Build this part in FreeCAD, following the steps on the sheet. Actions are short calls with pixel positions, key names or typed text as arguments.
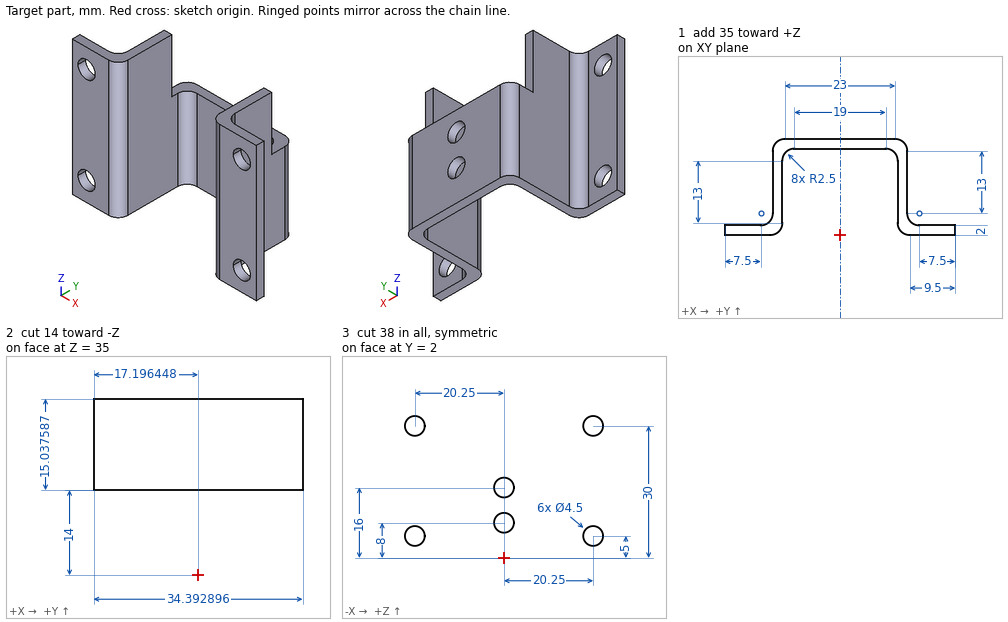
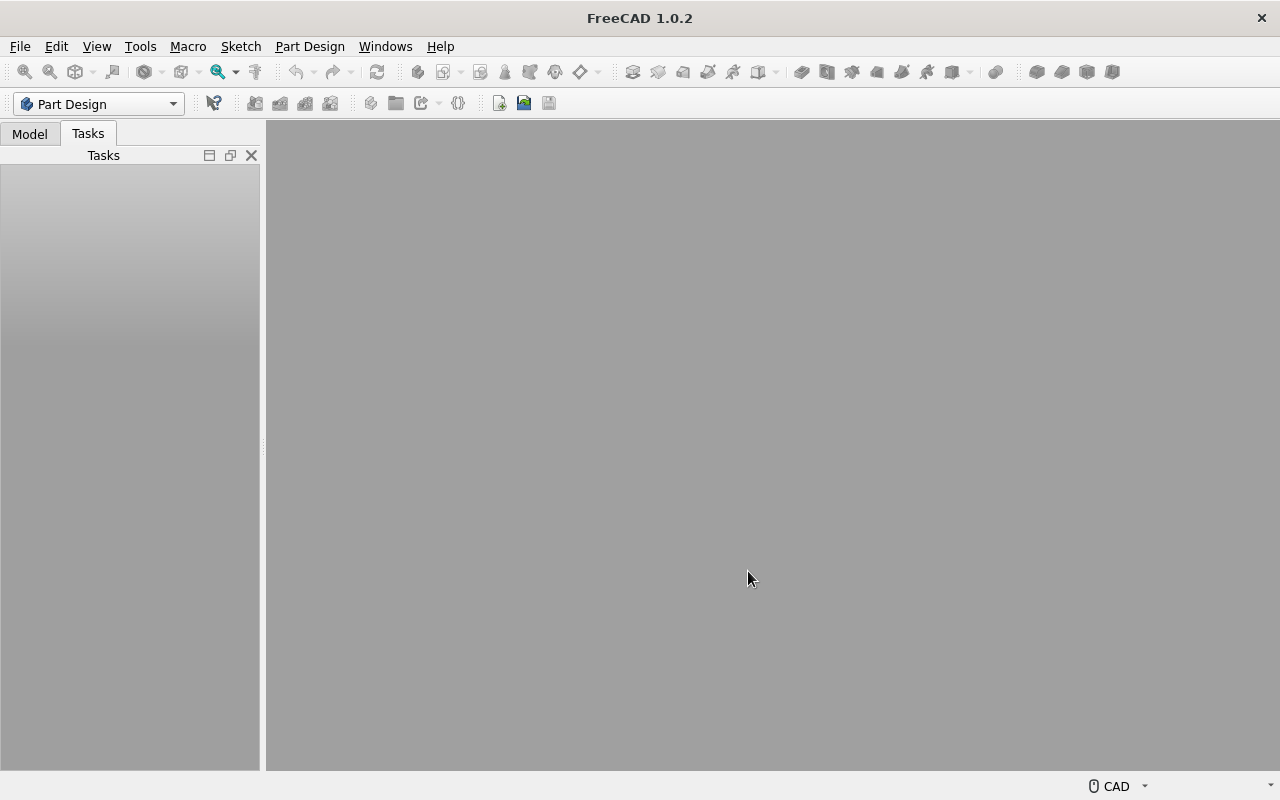
key(ctrl+n)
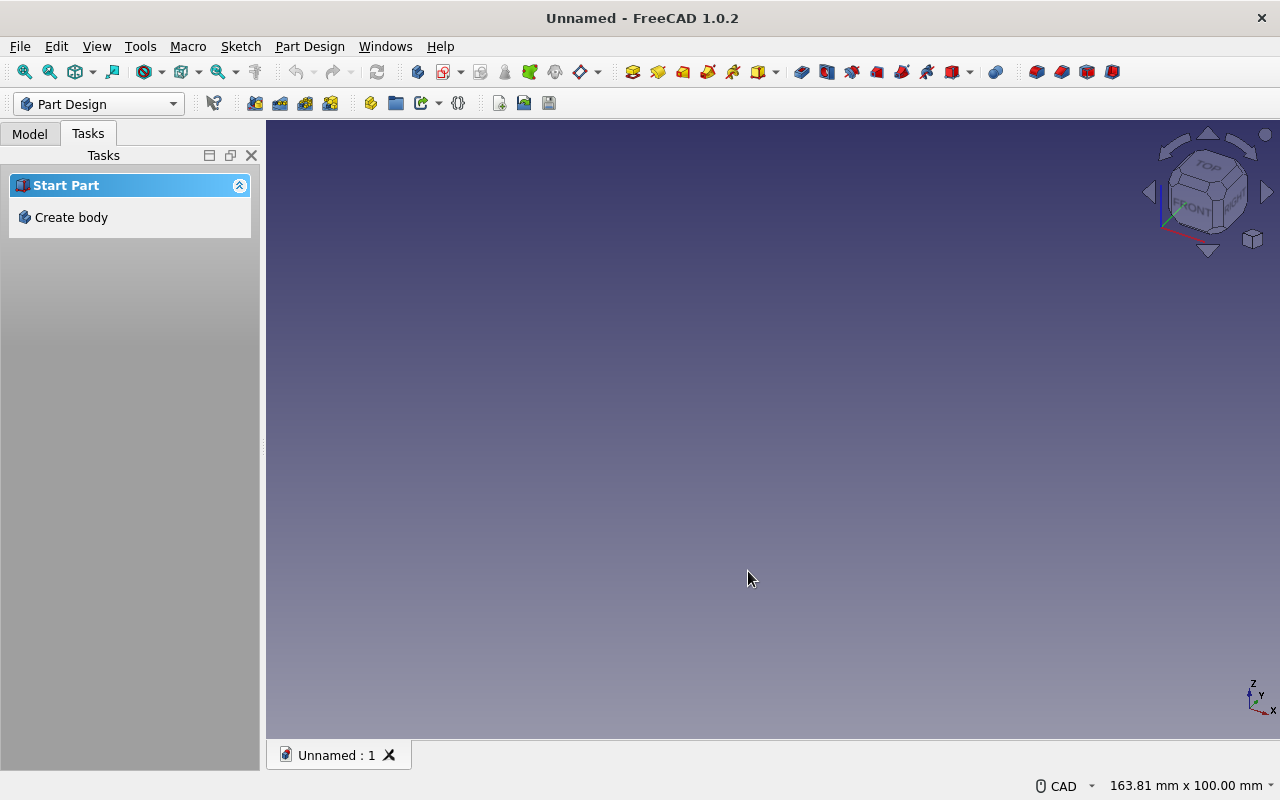
click(442, 72)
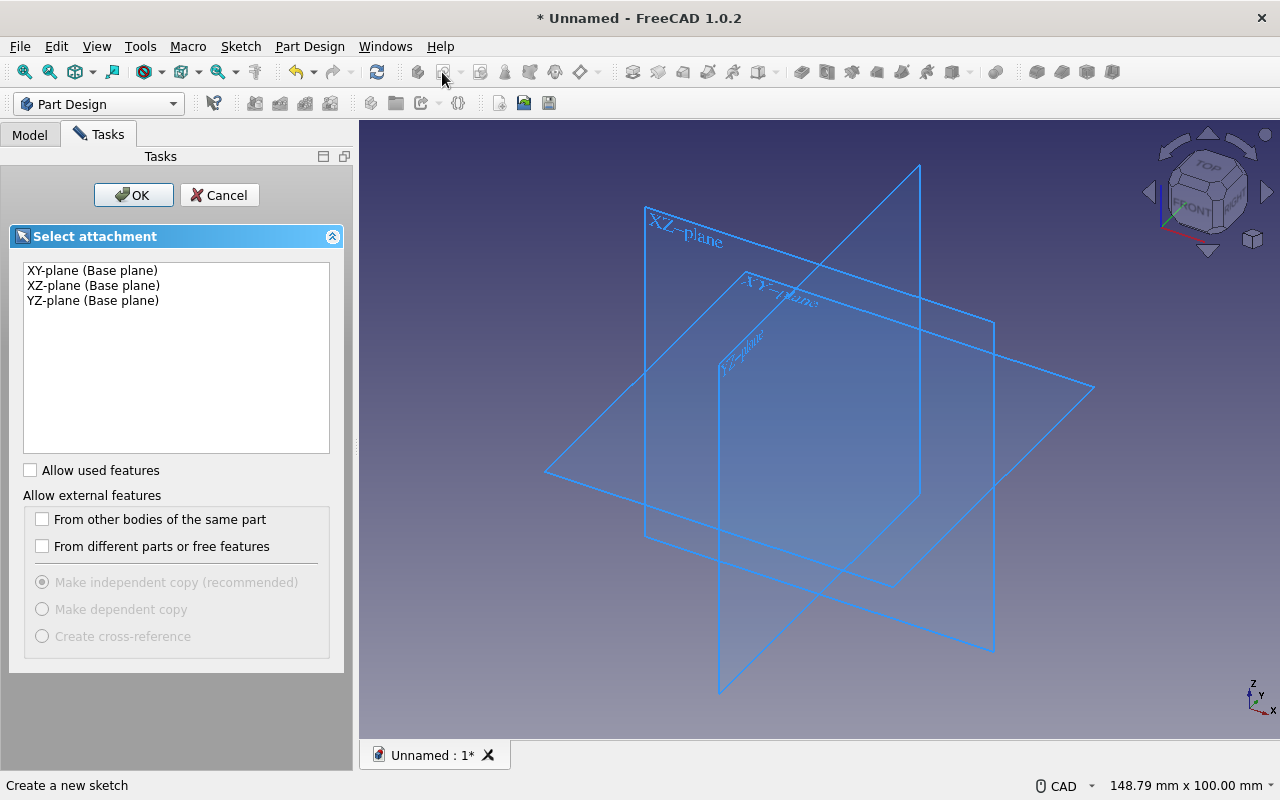
click(84, 270)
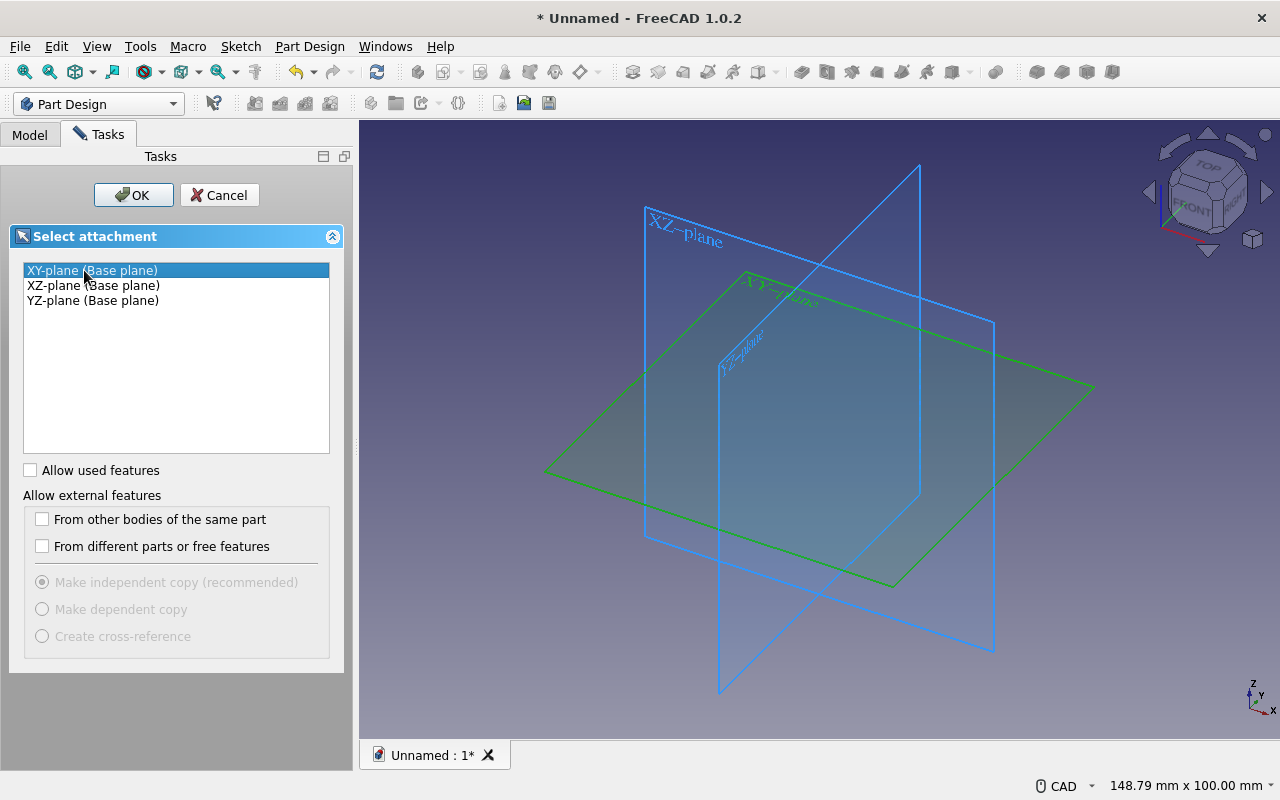
click(134, 195)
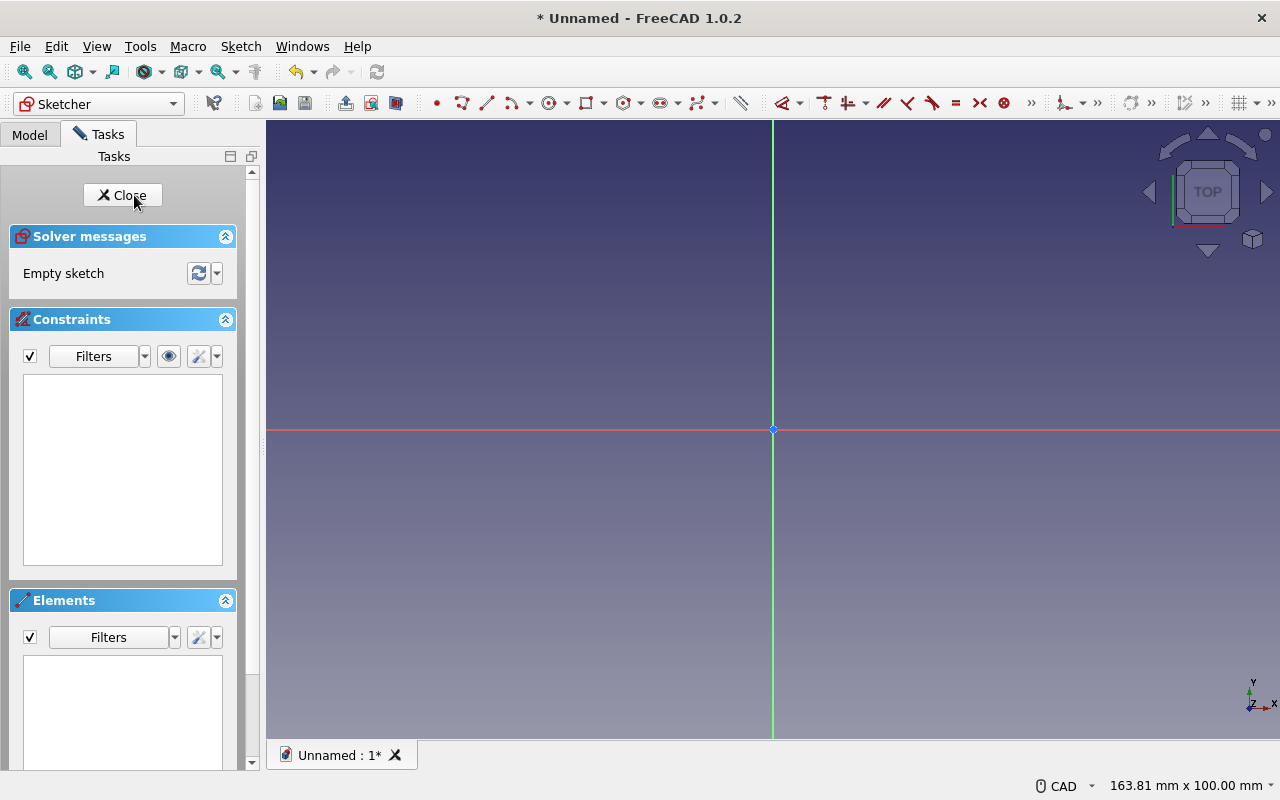
scroll(856, 292, up, 3)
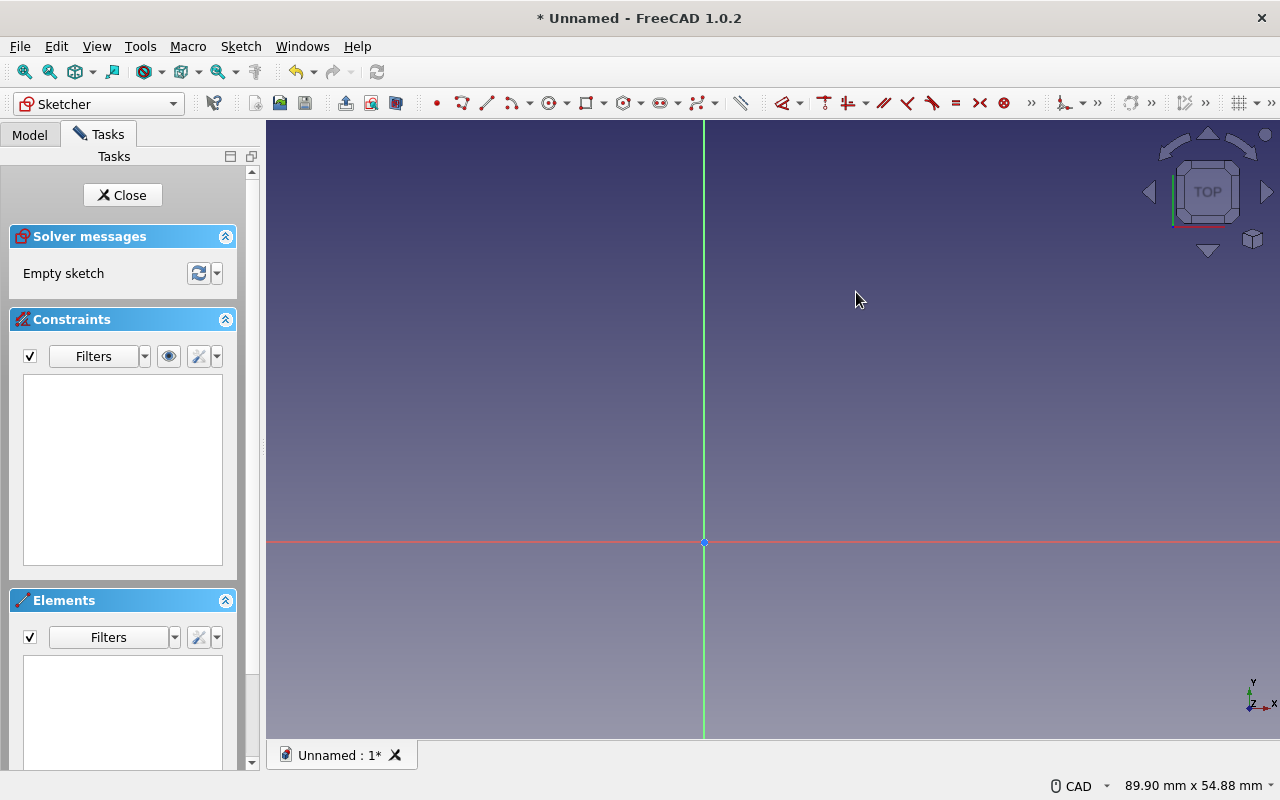
click(487, 104)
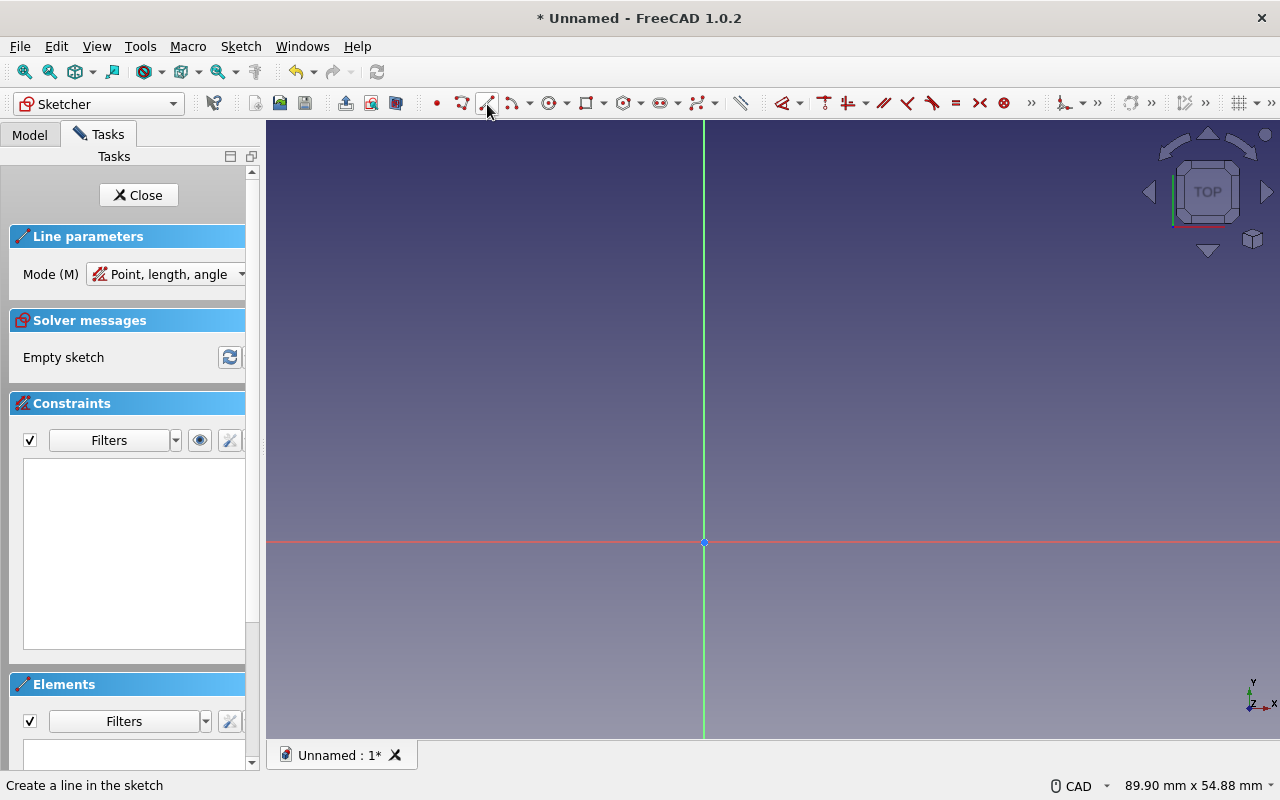
click(569, 514)
click(569, 367)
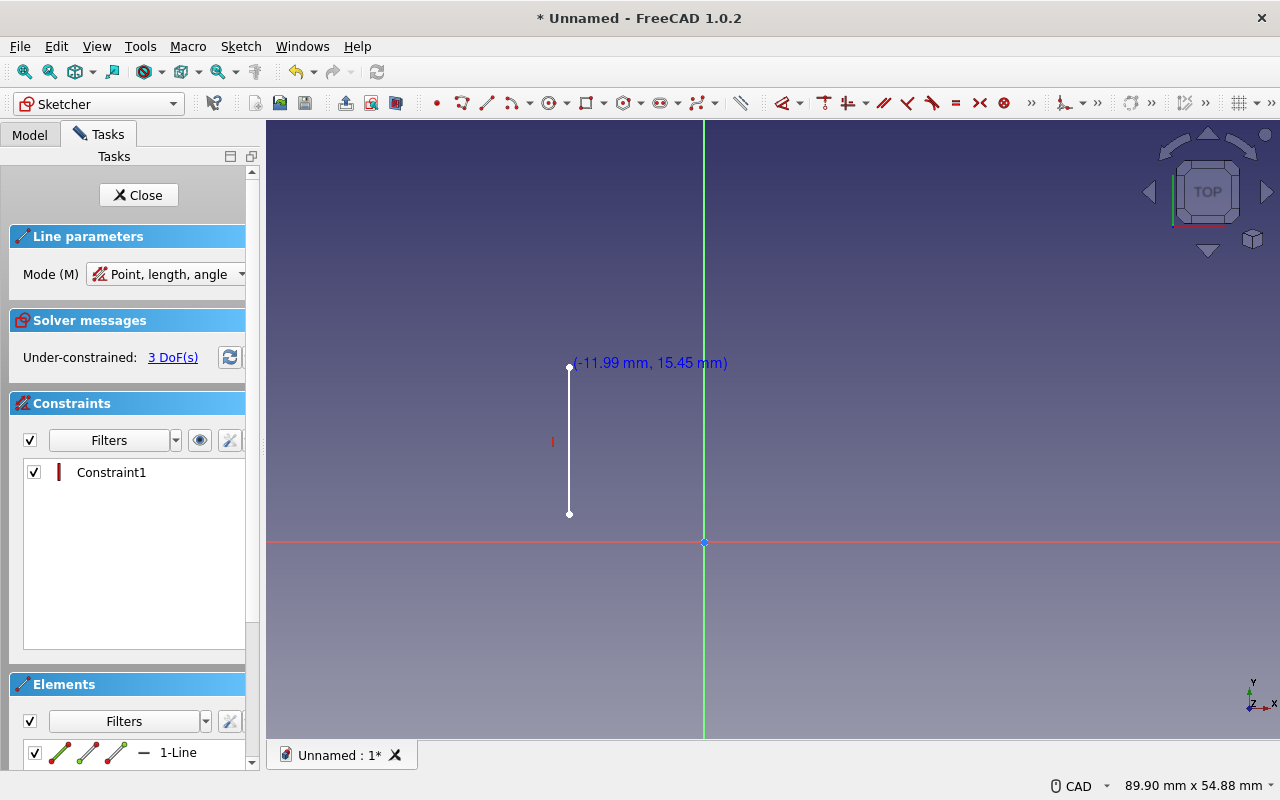
click(597, 339)
click(811, 339)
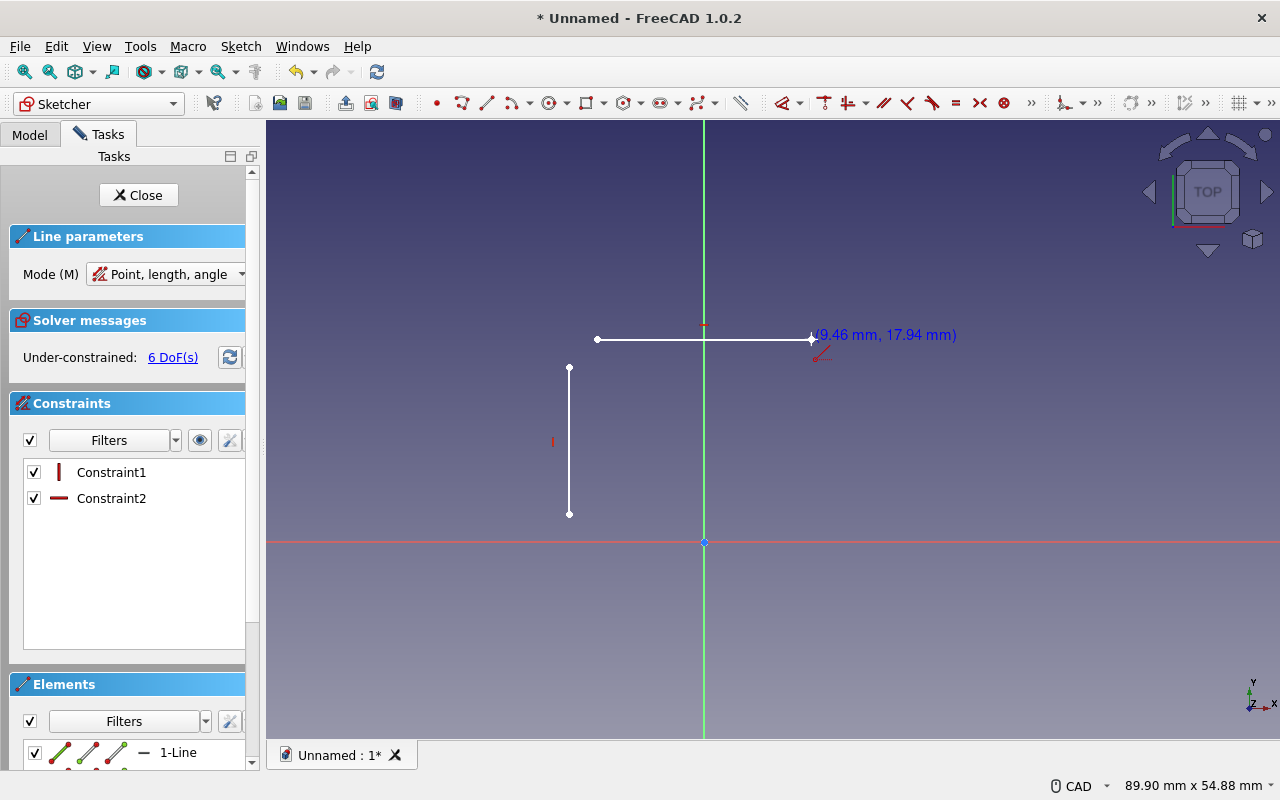
click(840, 367)
click(840, 514)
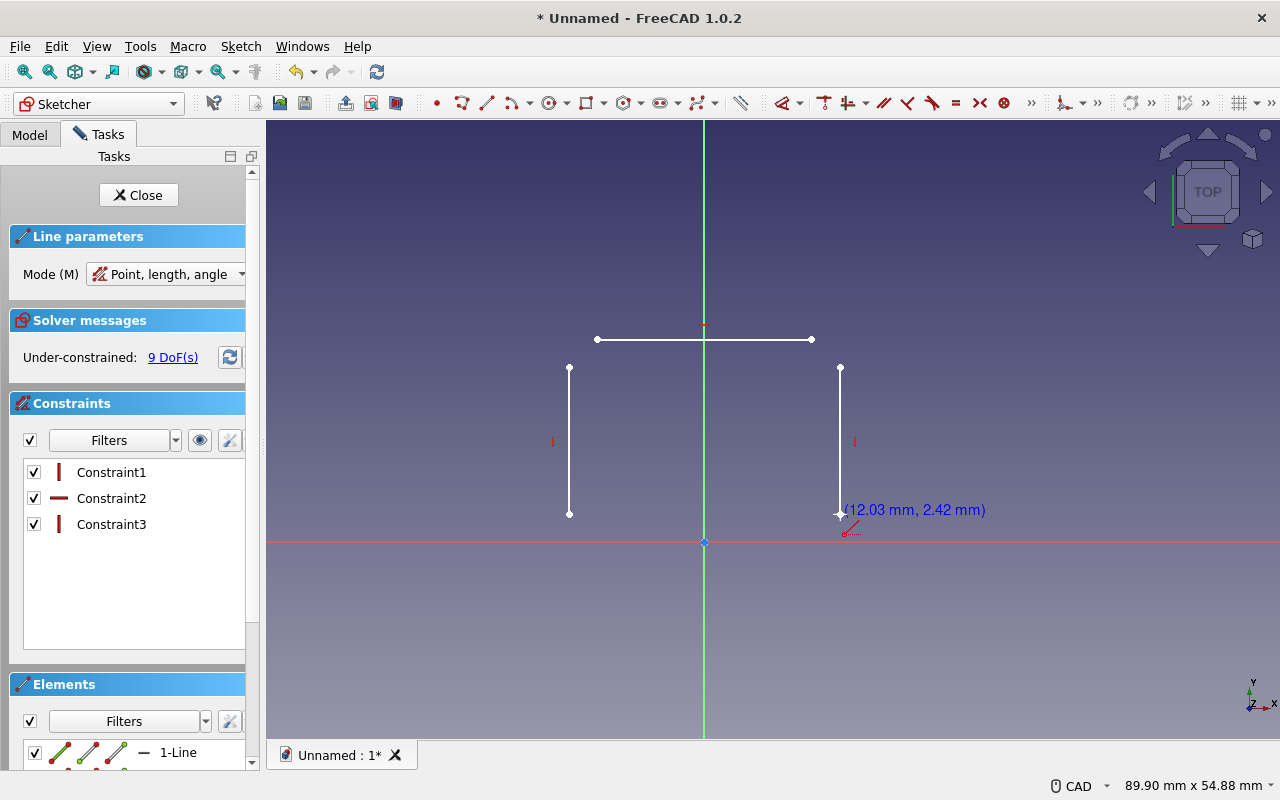
click(462, 104)